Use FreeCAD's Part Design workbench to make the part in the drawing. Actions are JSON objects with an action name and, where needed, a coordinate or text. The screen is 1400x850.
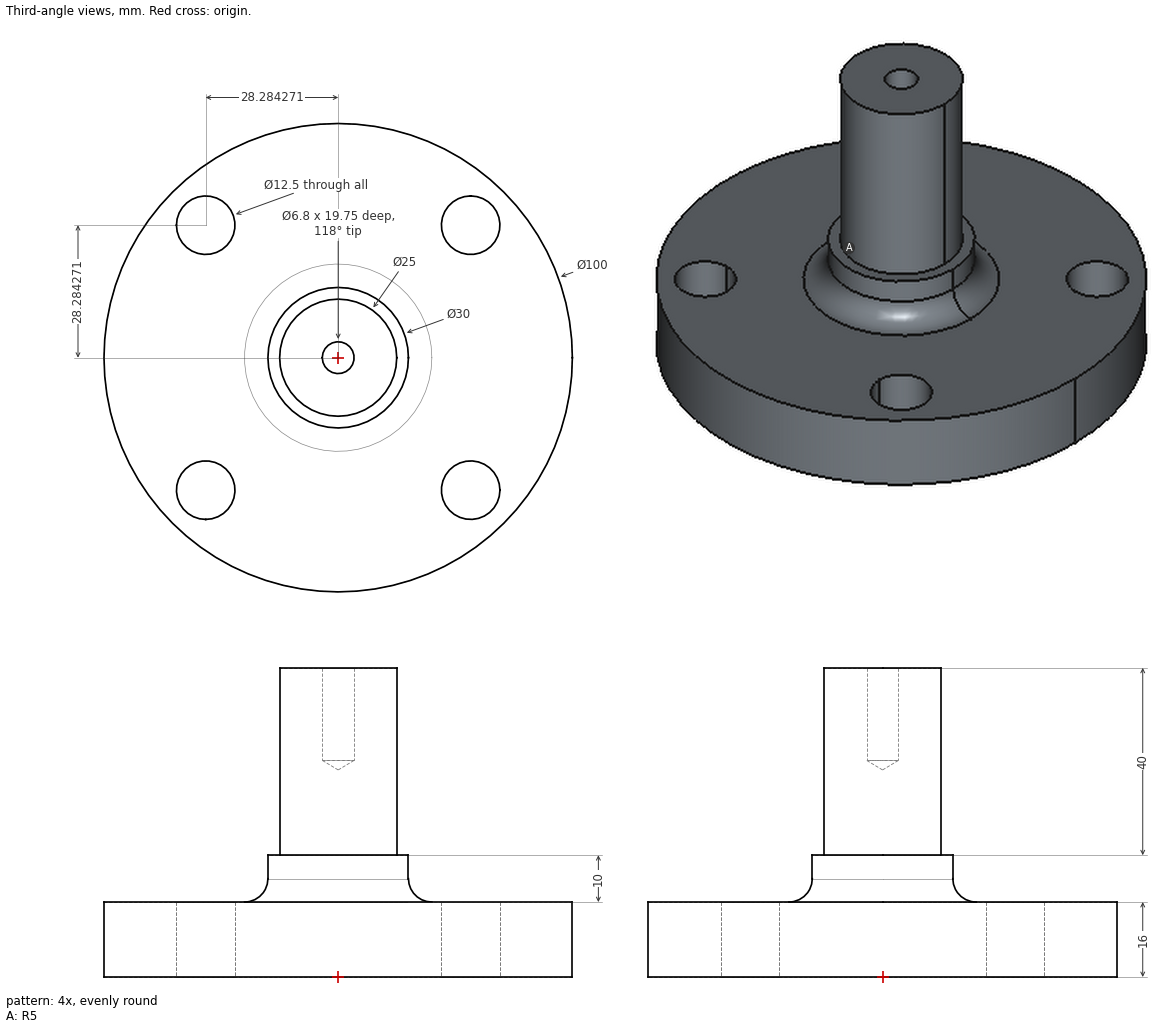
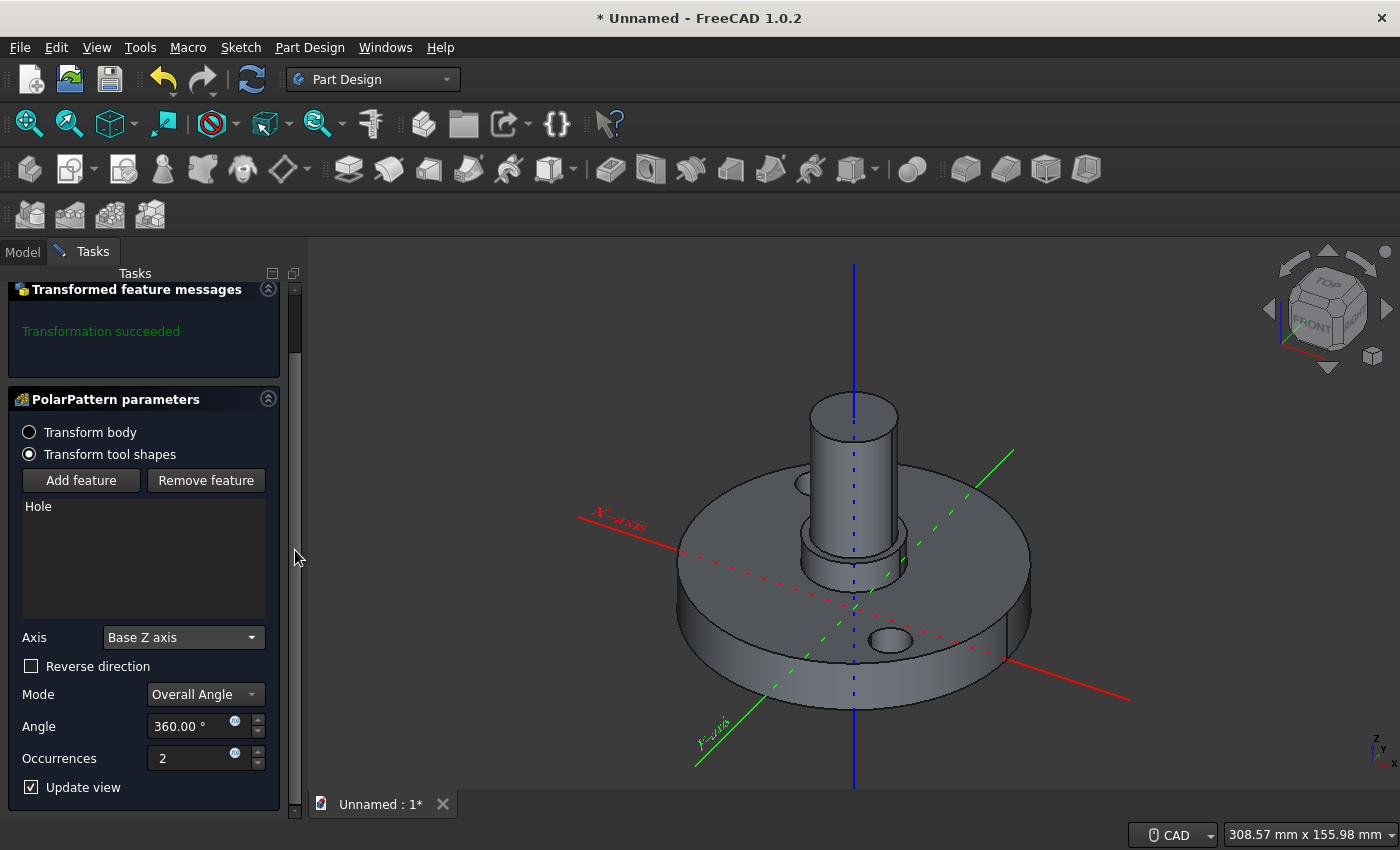
{"action": "triple_click", "coordinate": [198, 758]}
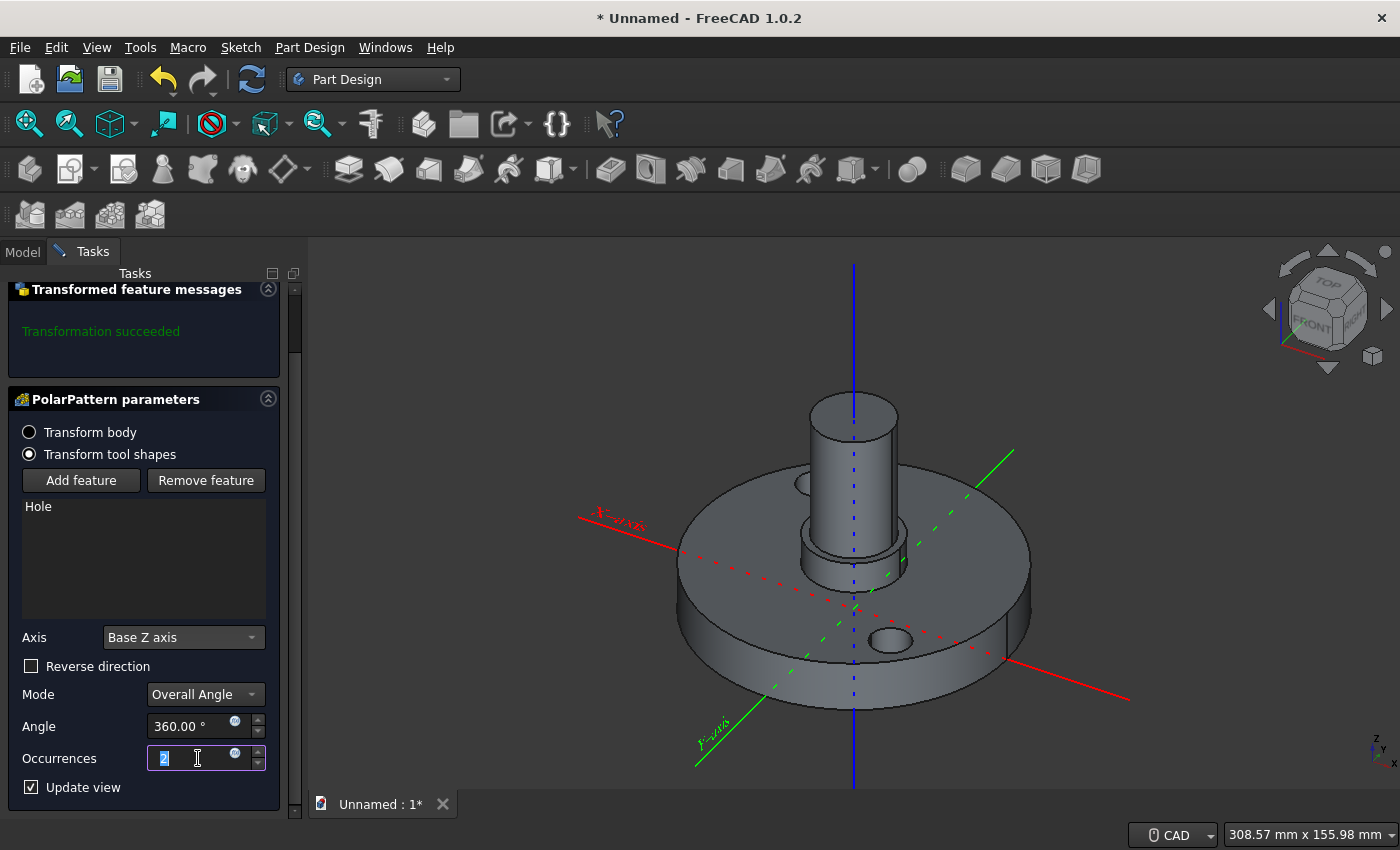
{"action": "type", "text": "4"}
{"action": "key", "text": "Tab"}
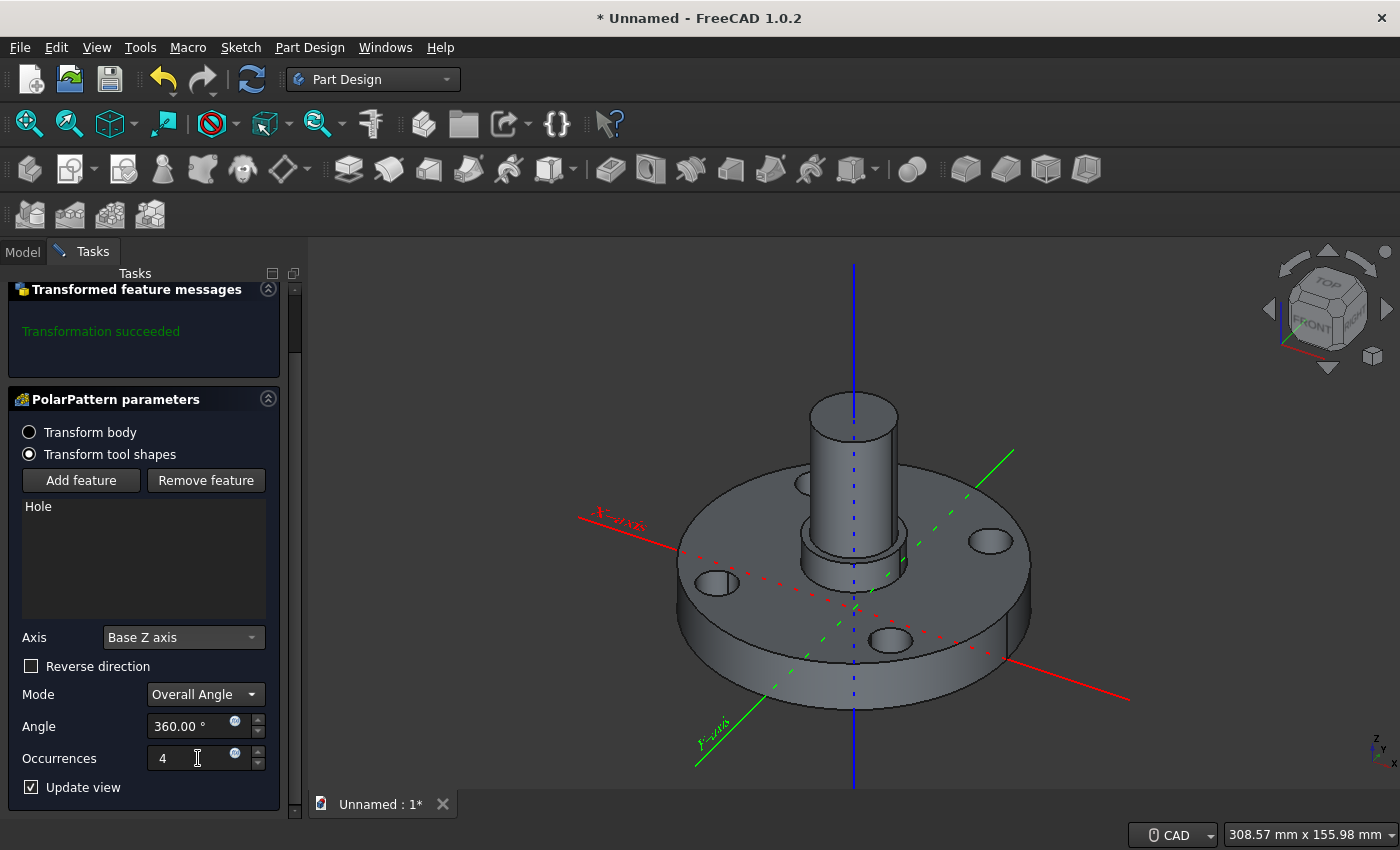
{"action": "scroll", "coordinate": [295, 550], "scroll_direction": "up", "scroll_amount": 2}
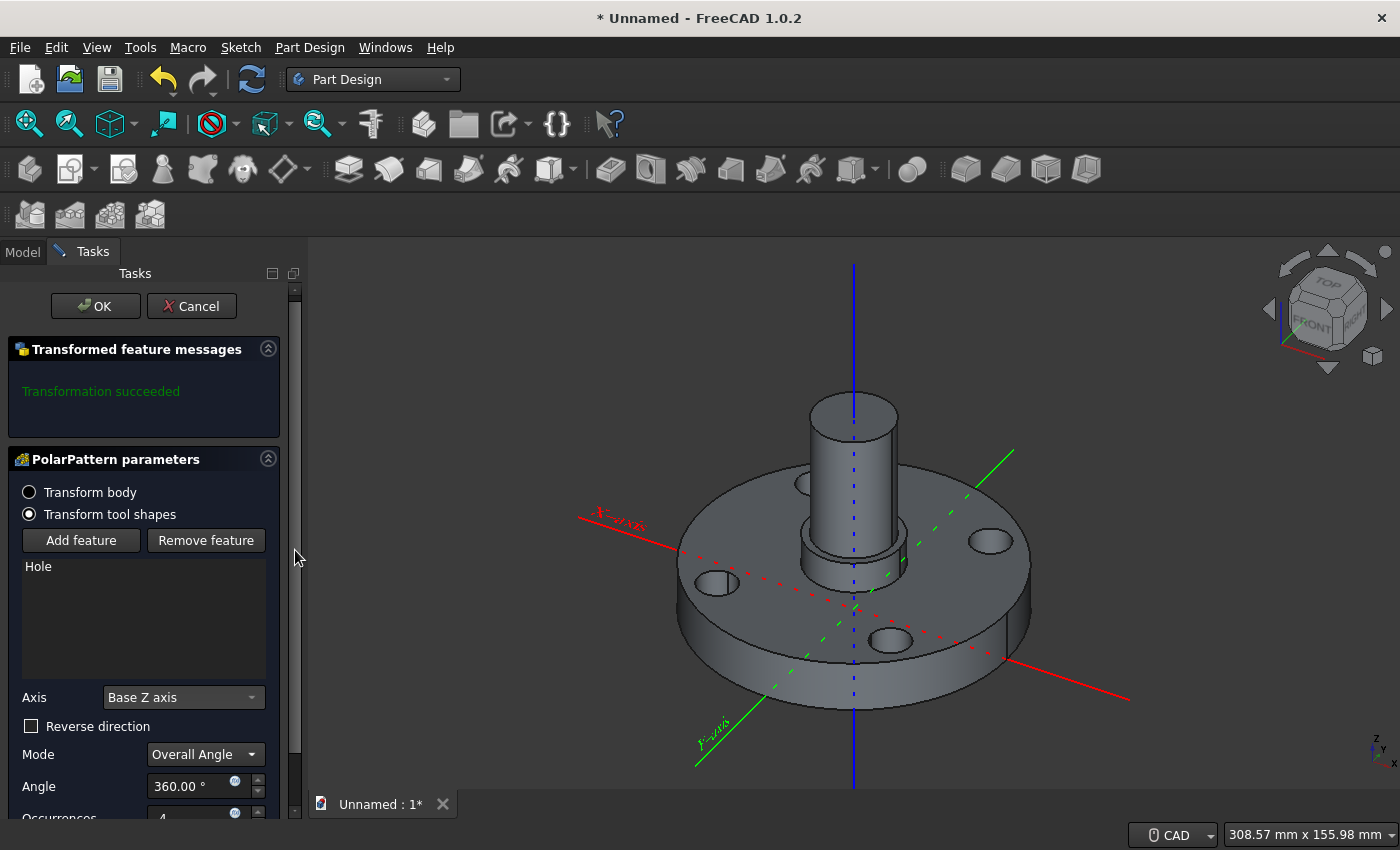
{"action": "left_click", "coordinate": [96, 312]}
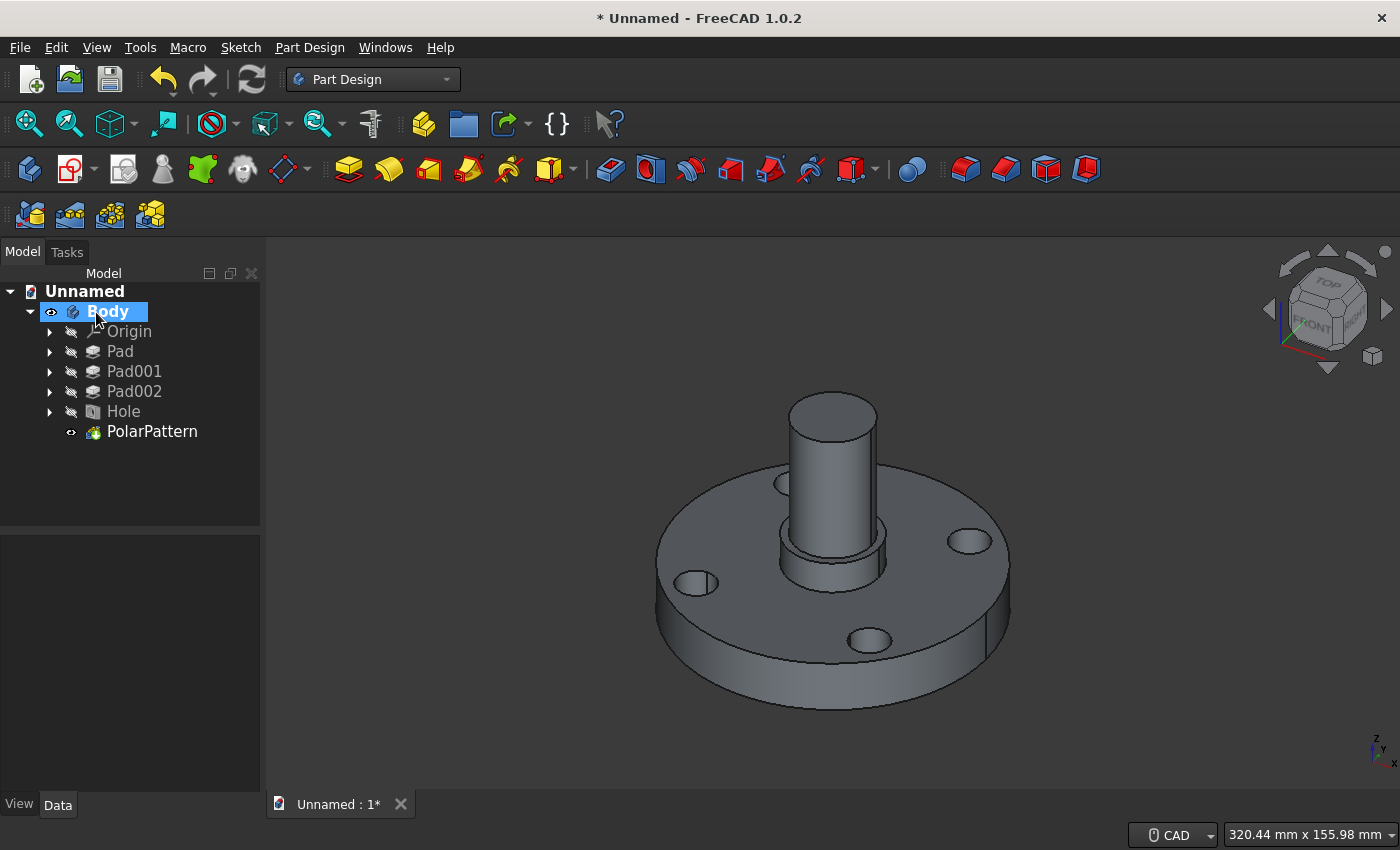
{"action": "left_click", "coordinate": [833, 416]}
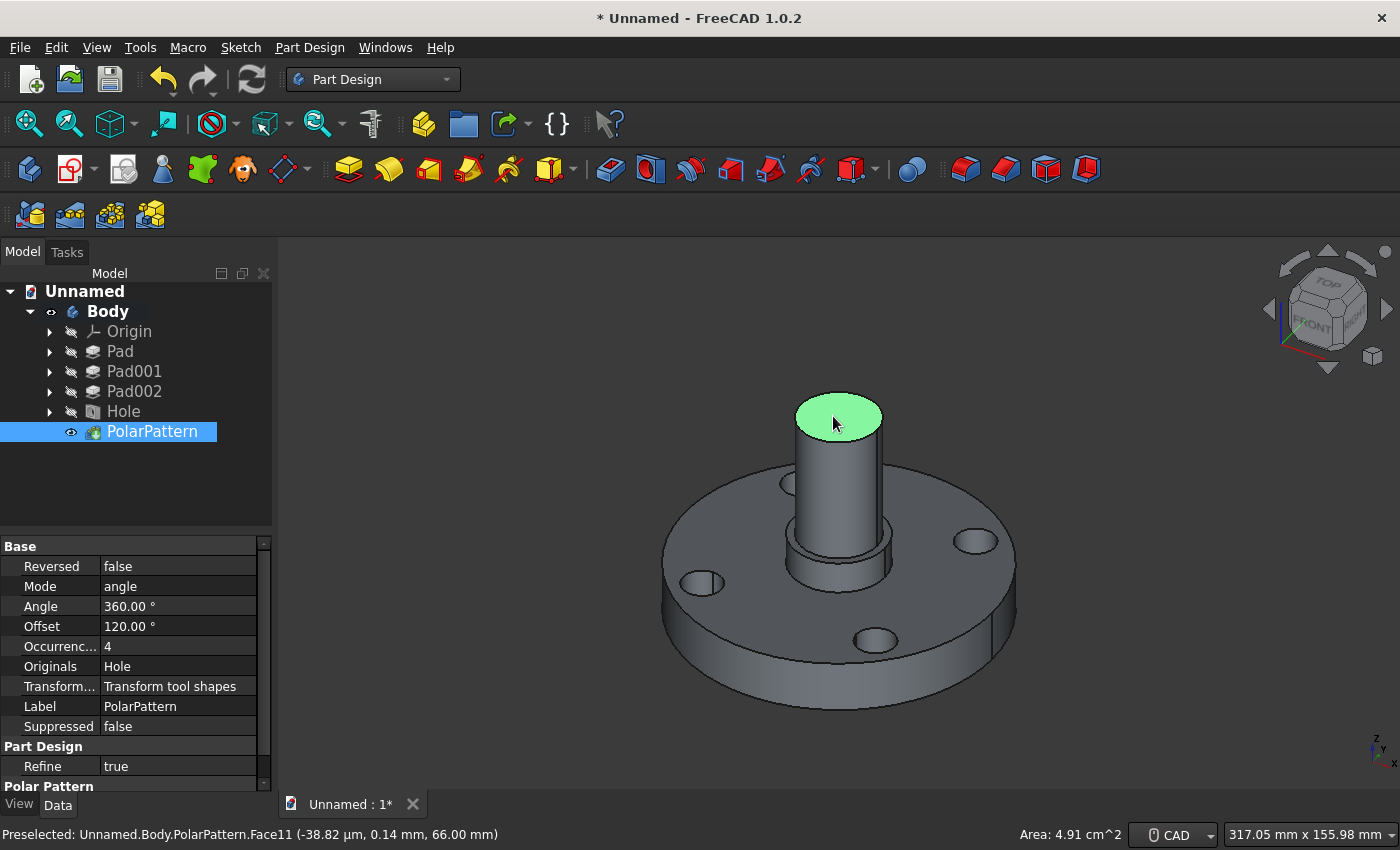
{"action": "left_click", "coordinate": [70, 170]}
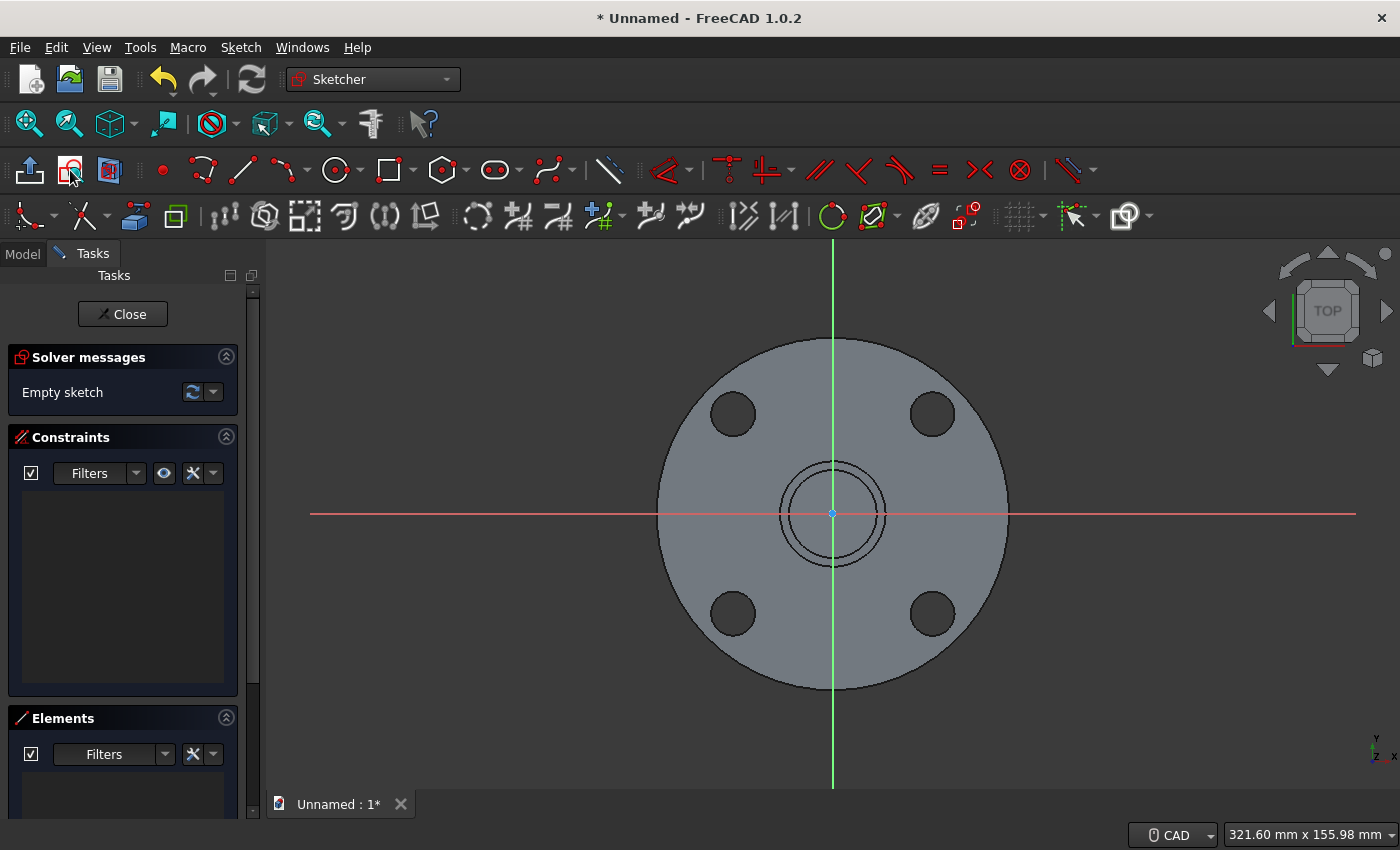
{"action": "scroll", "coordinate": [838, 514], "scroll_direction": "up", "scroll_amount": 13}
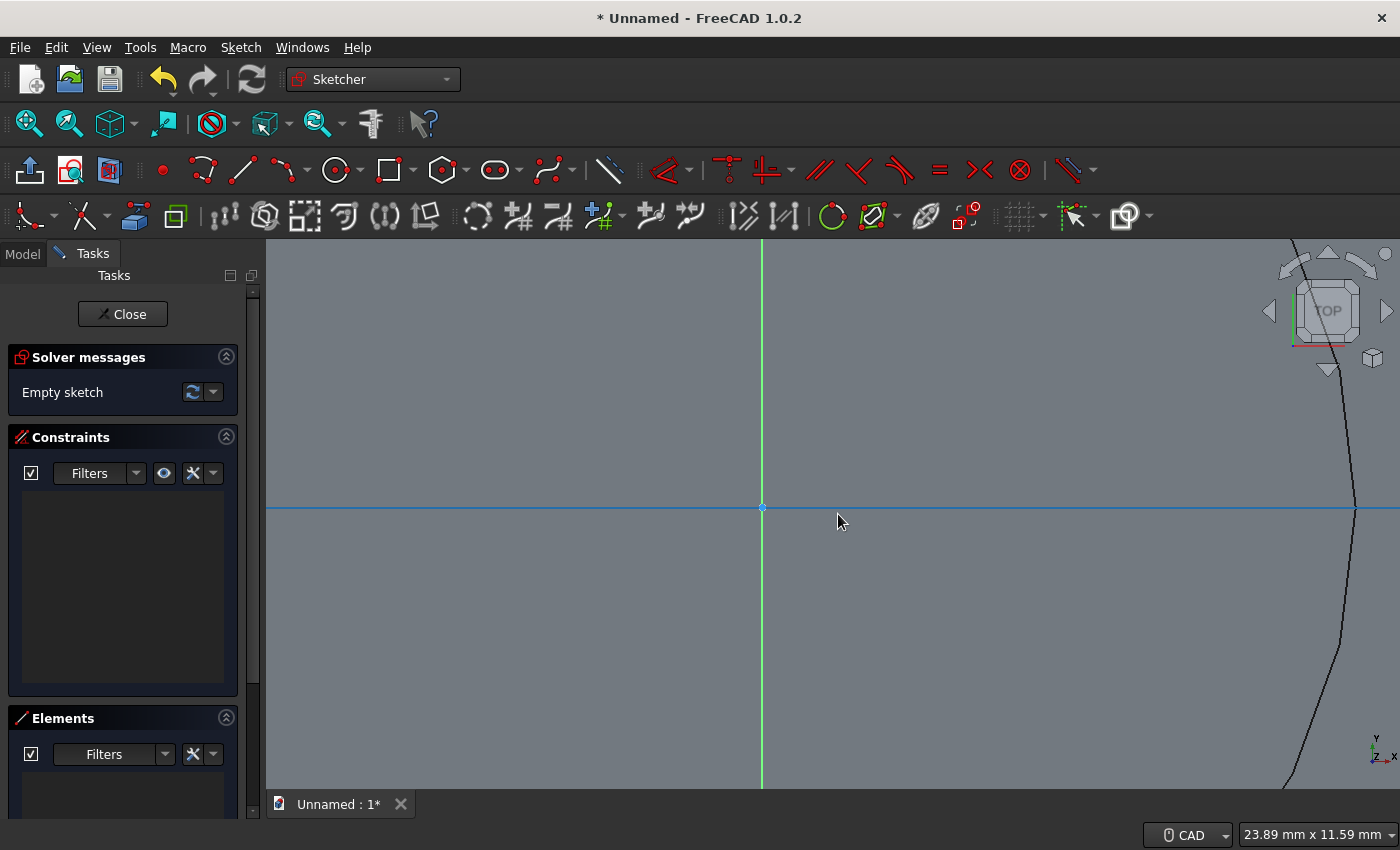
{"action": "key", "text": "g c"}